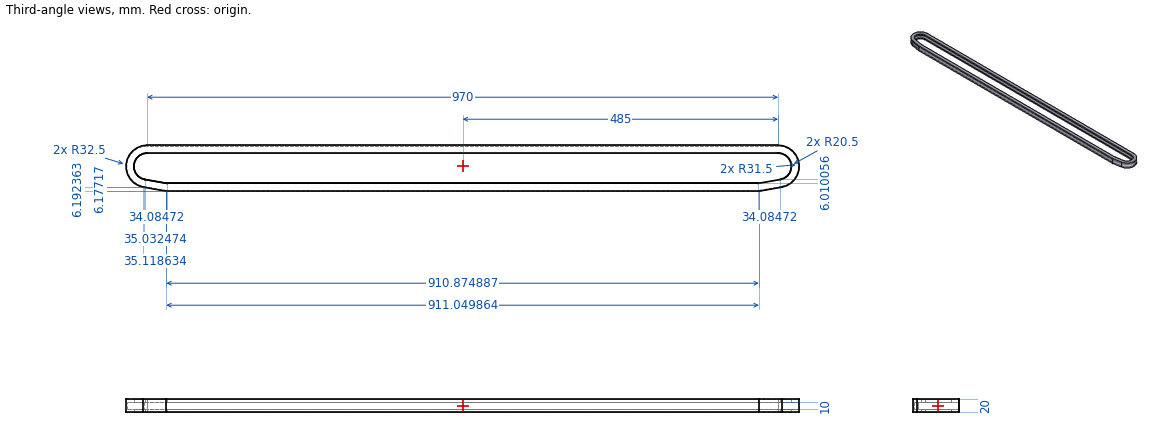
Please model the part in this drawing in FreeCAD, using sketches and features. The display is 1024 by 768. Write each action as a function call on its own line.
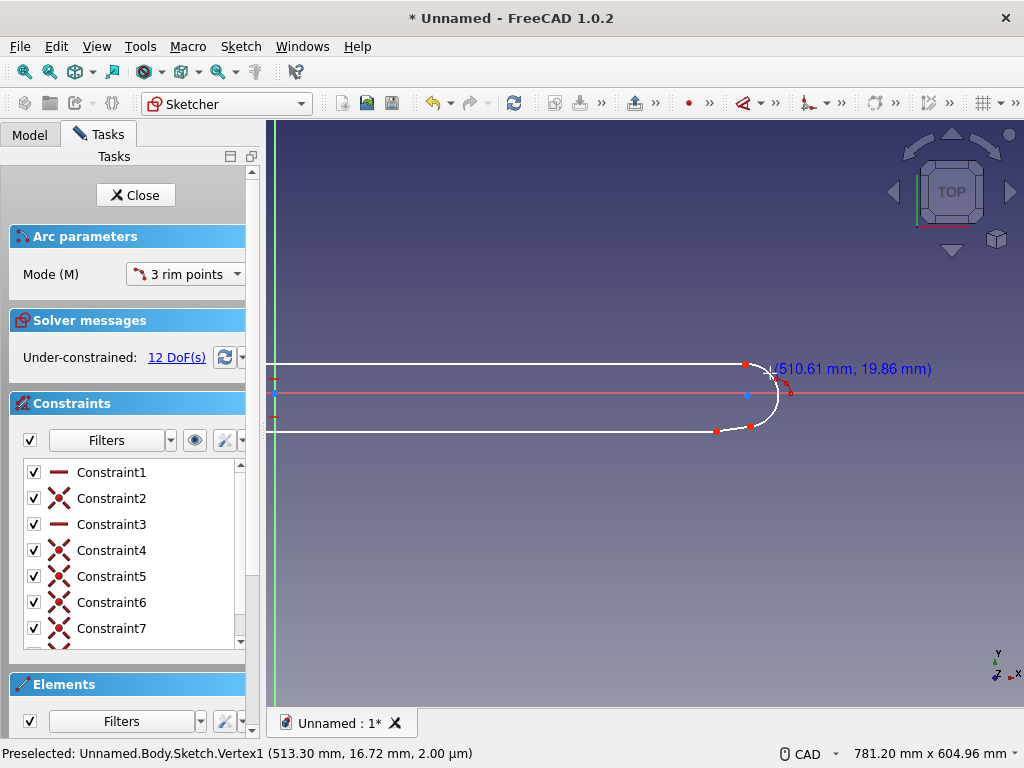
key(g)
key(l)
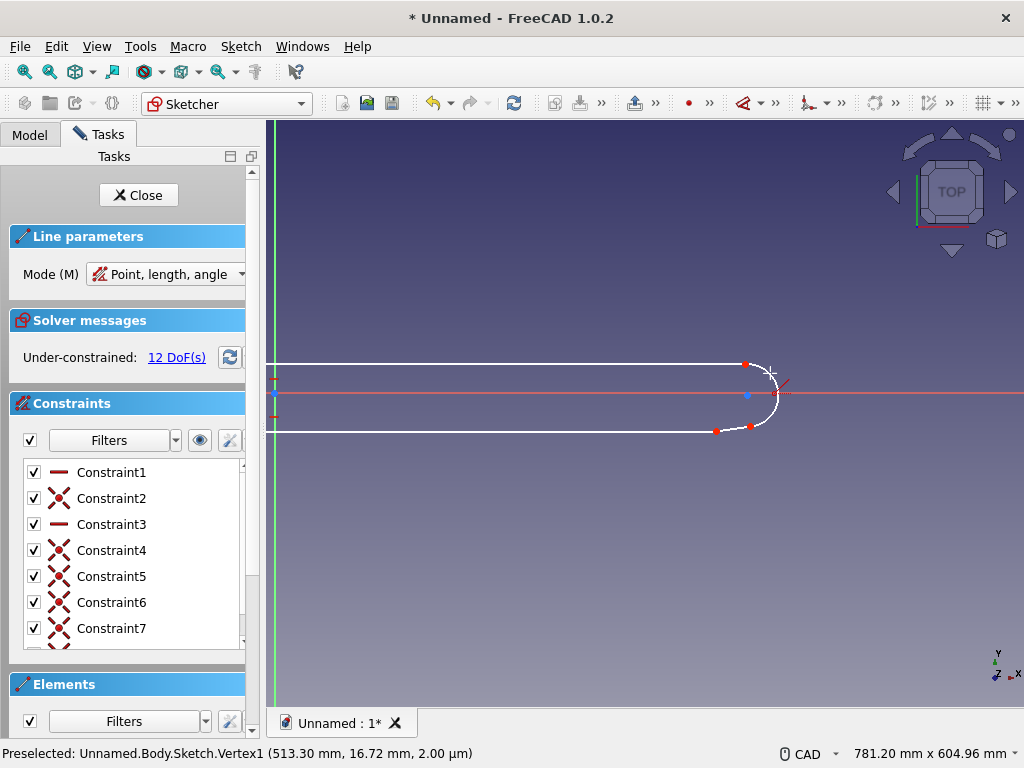
scroll(752, 424, down, 5)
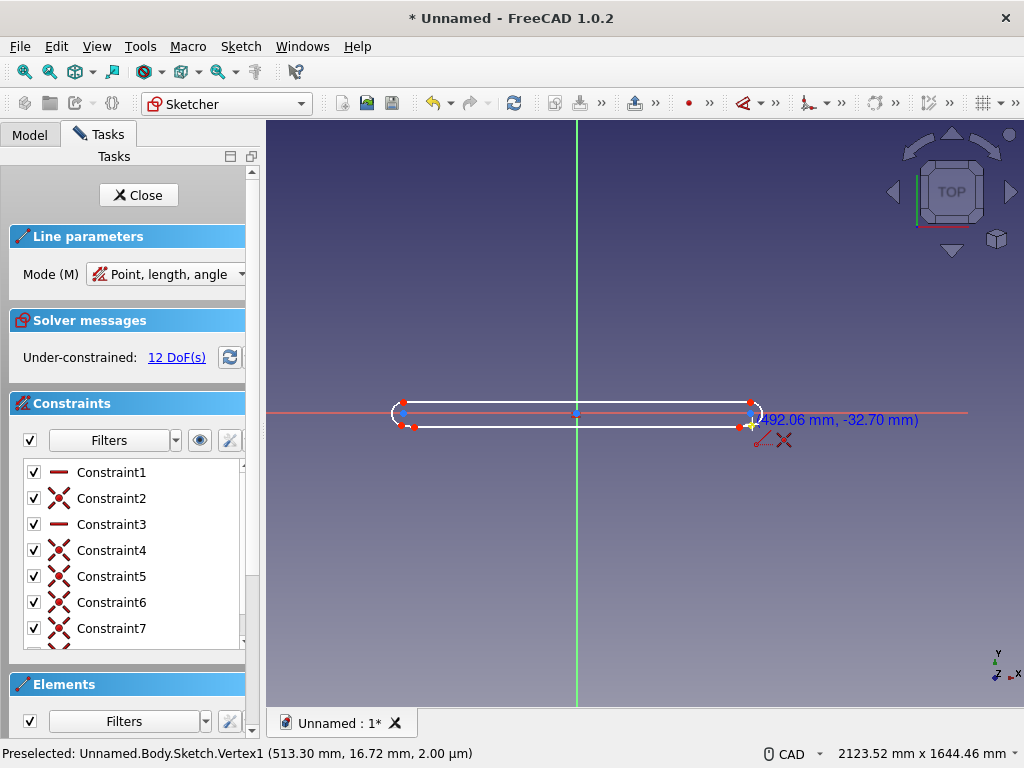
scroll(404, 406, up, 7)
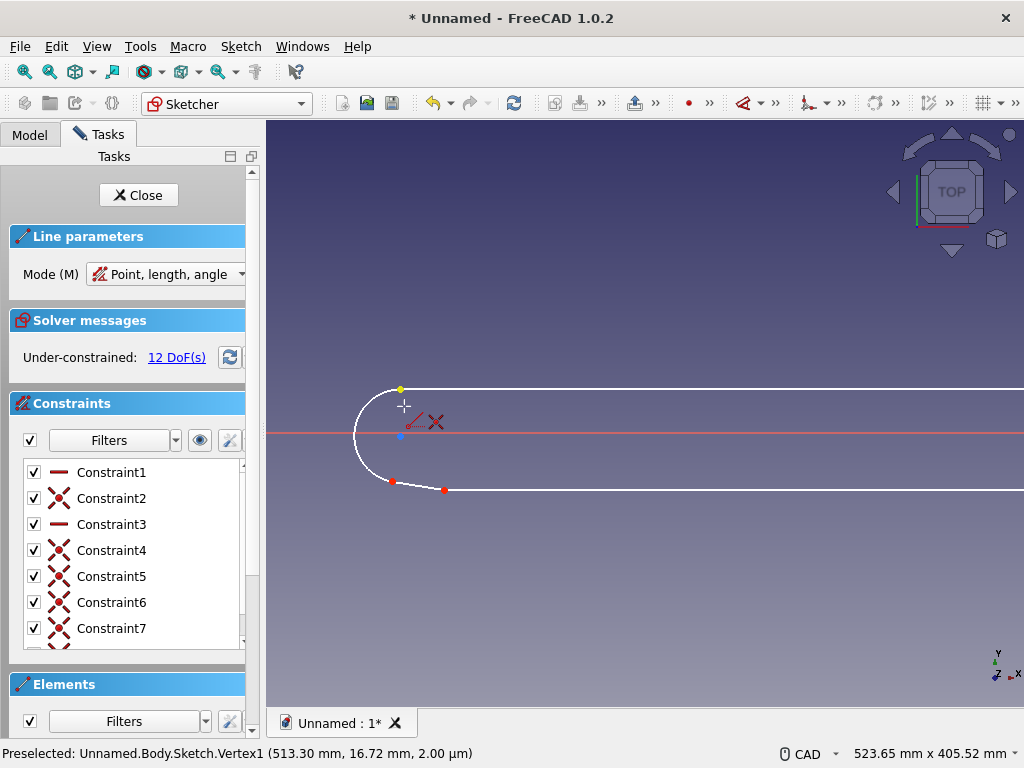
click(402, 403)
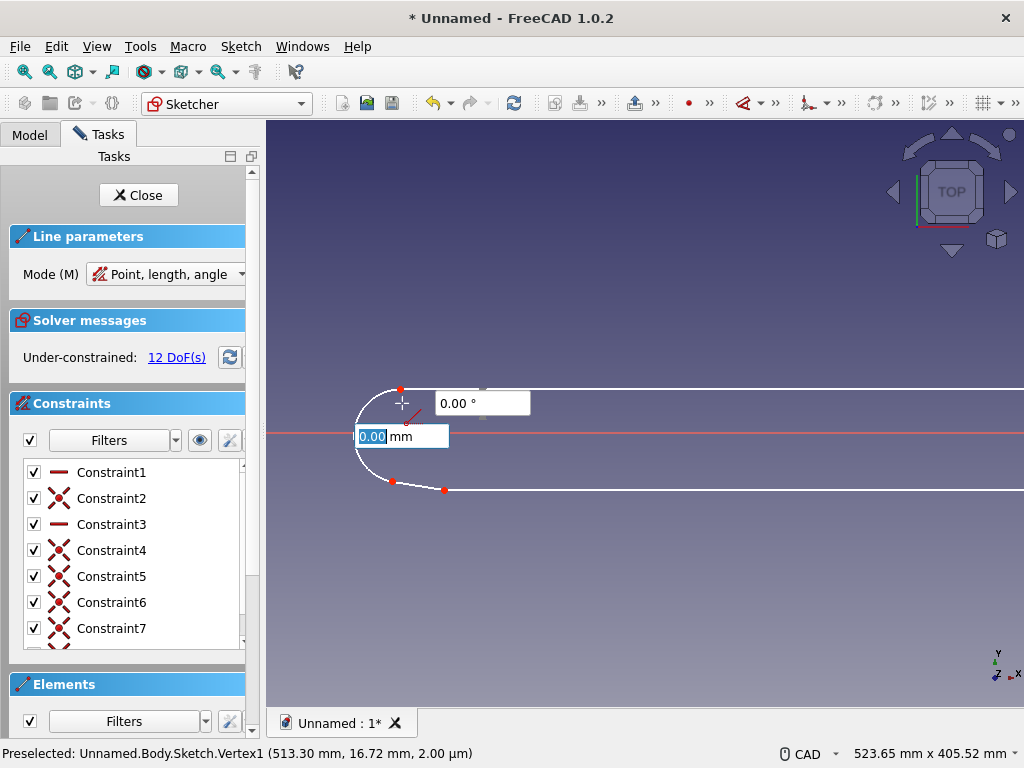
scroll(404, 406, down, 7)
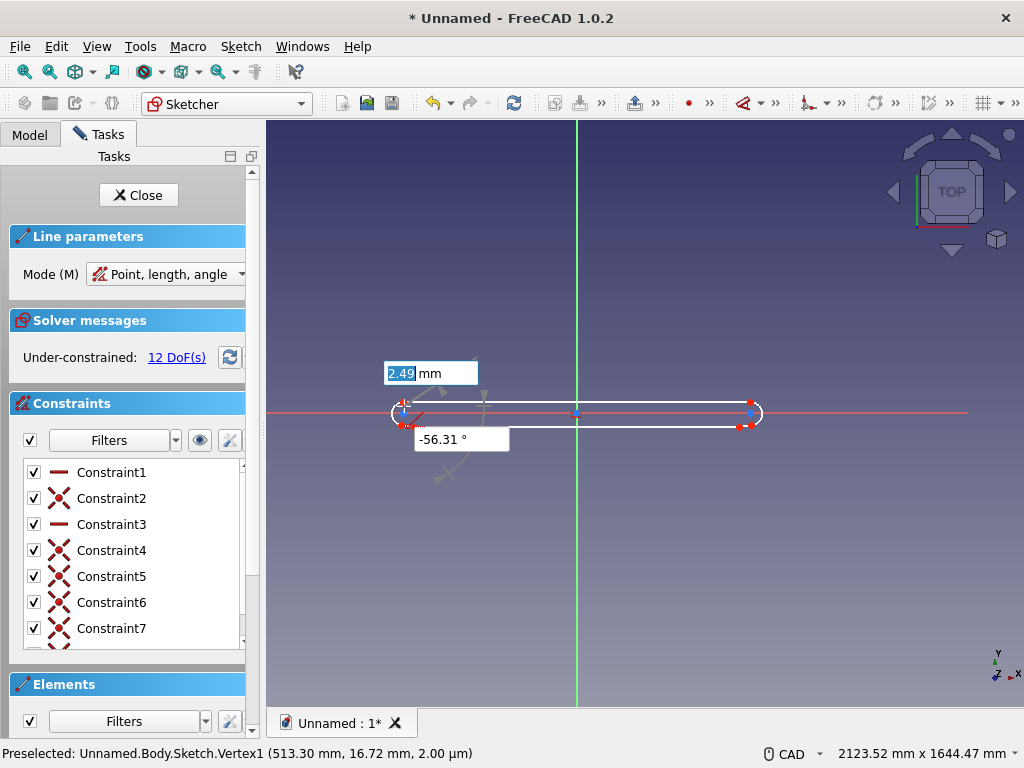
scroll(750, 406, up, 7)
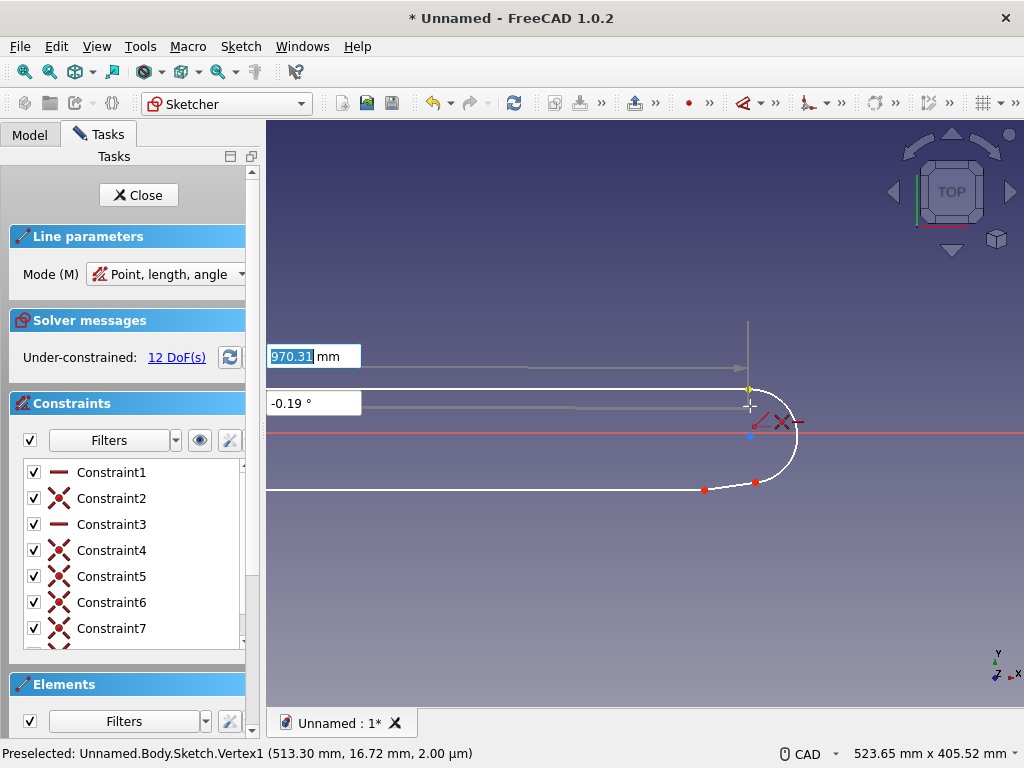
click(748, 403)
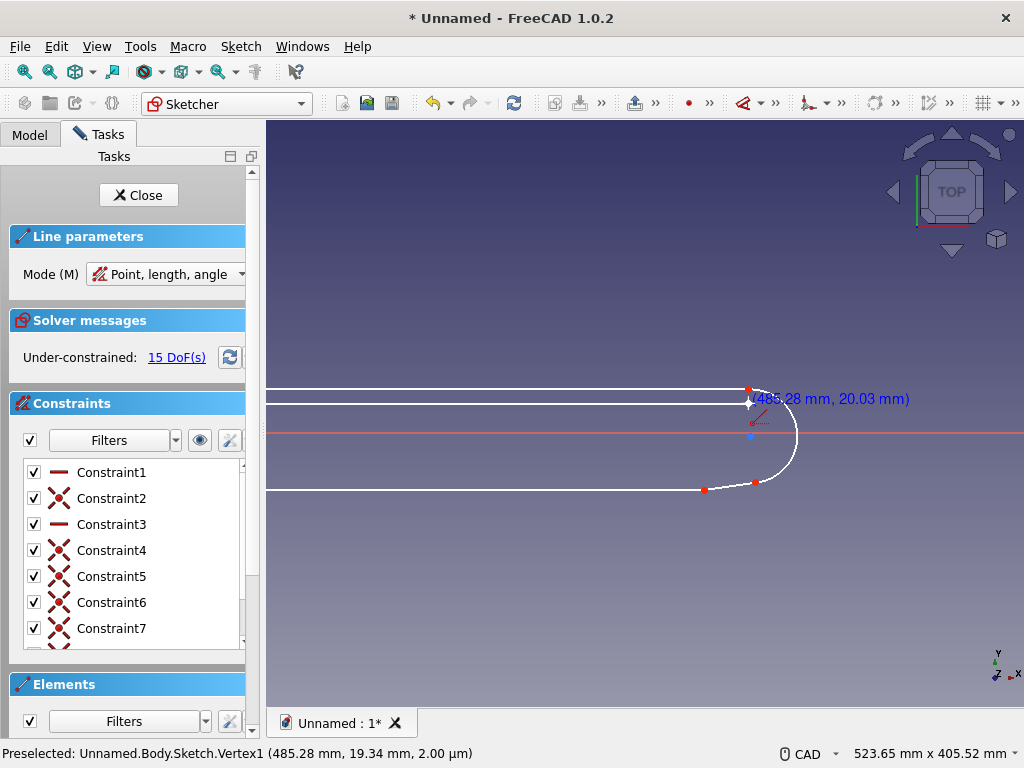
key(g)
key(m)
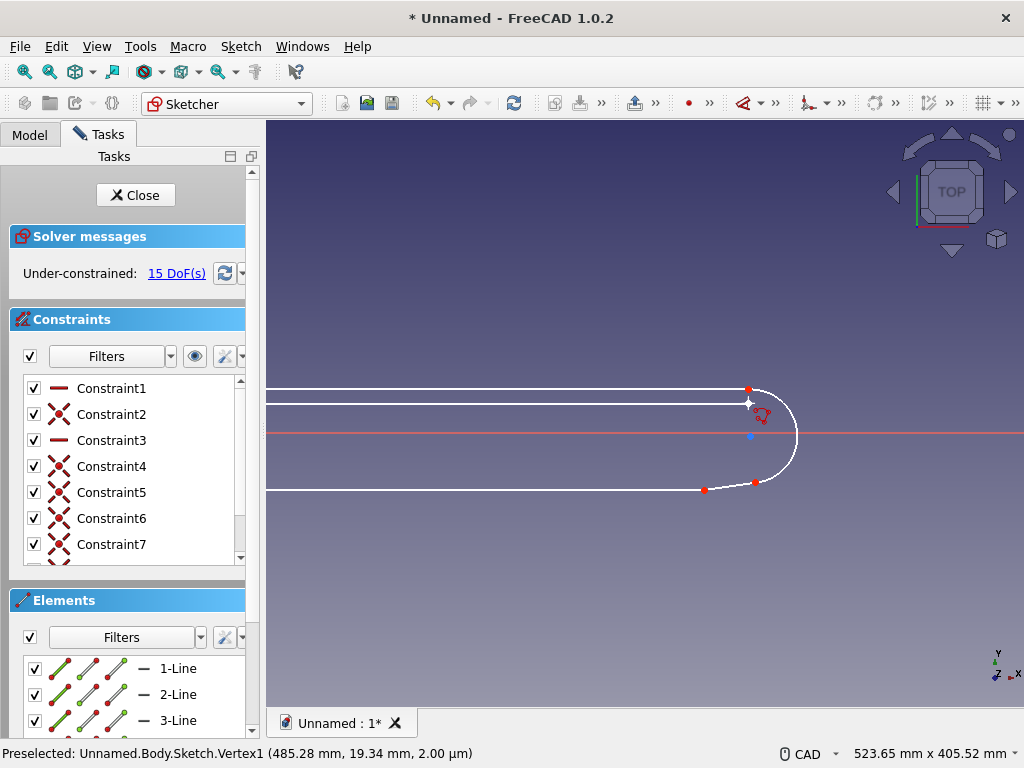
click(753, 462)
click(703, 471)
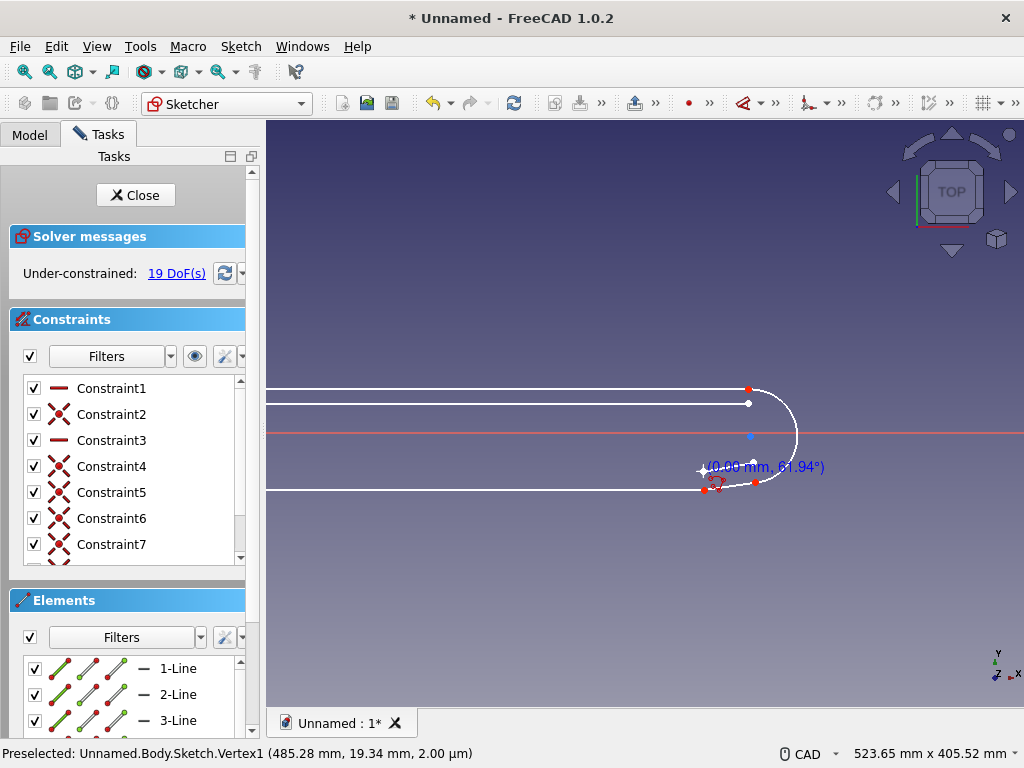
scroll(750, 406, down, 7)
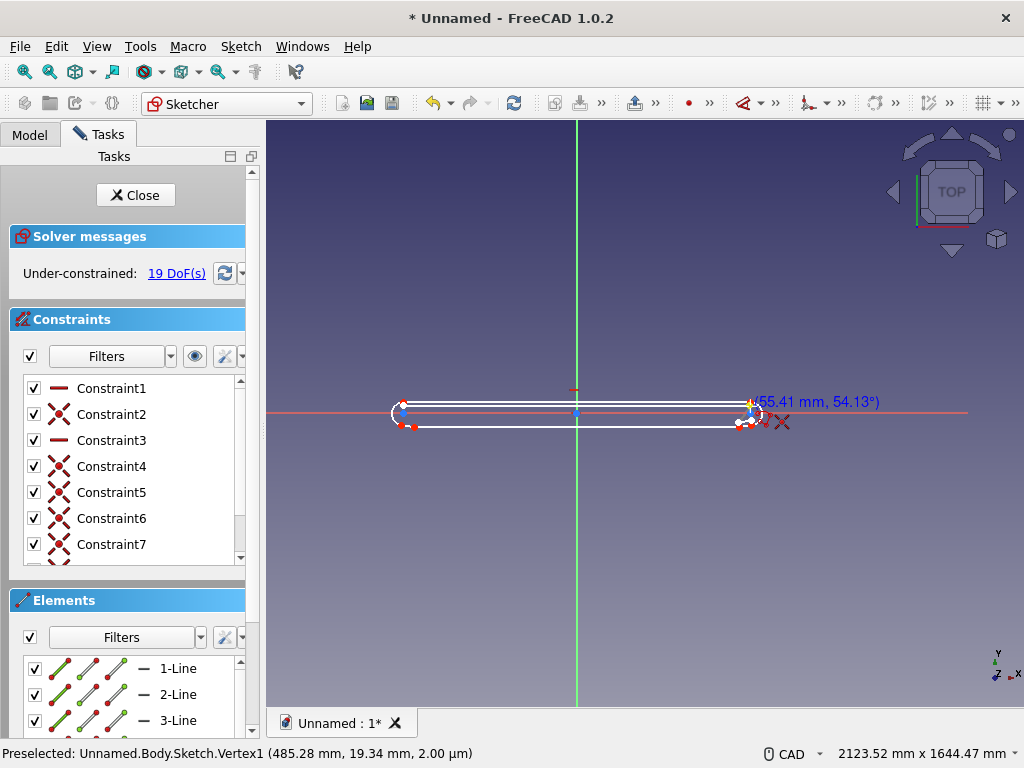
scroll(415, 422, up, 7)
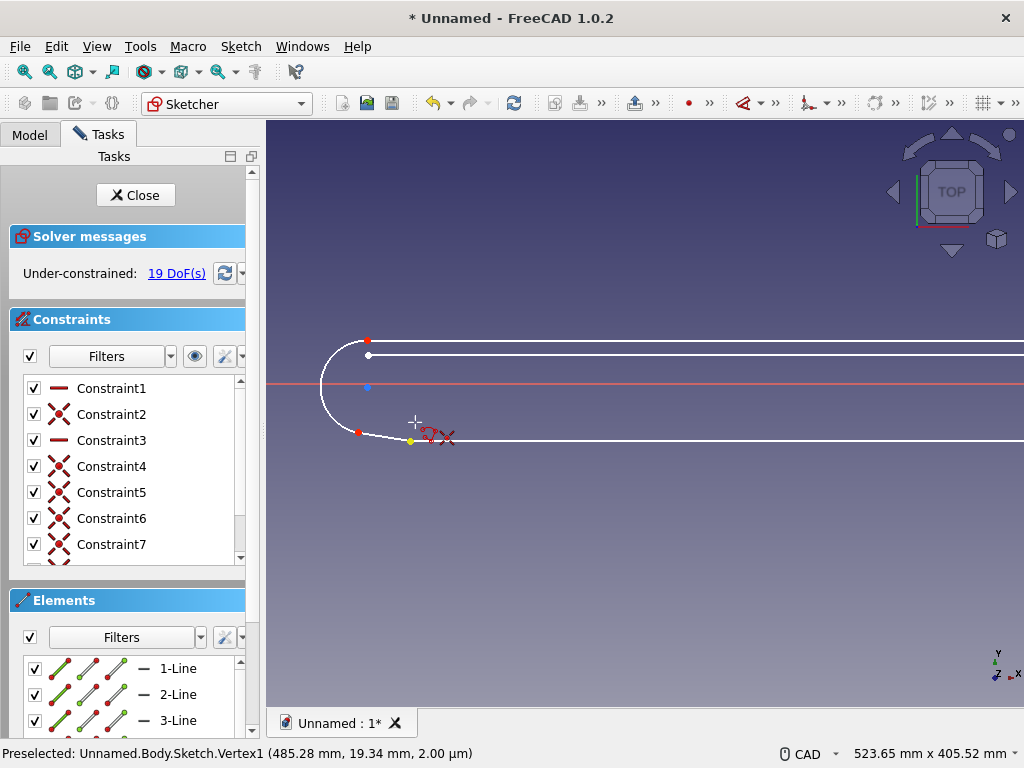
click(413, 422)
click(363, 413)
right_click(363, 413)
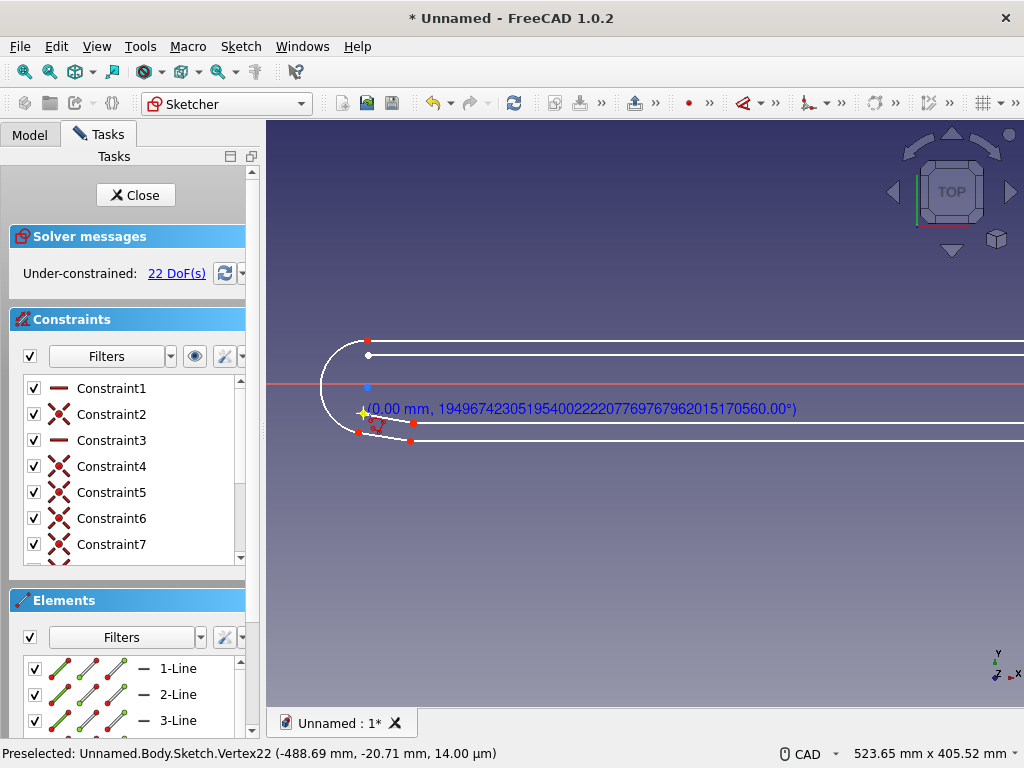
key(g)
key(3)
key(a)